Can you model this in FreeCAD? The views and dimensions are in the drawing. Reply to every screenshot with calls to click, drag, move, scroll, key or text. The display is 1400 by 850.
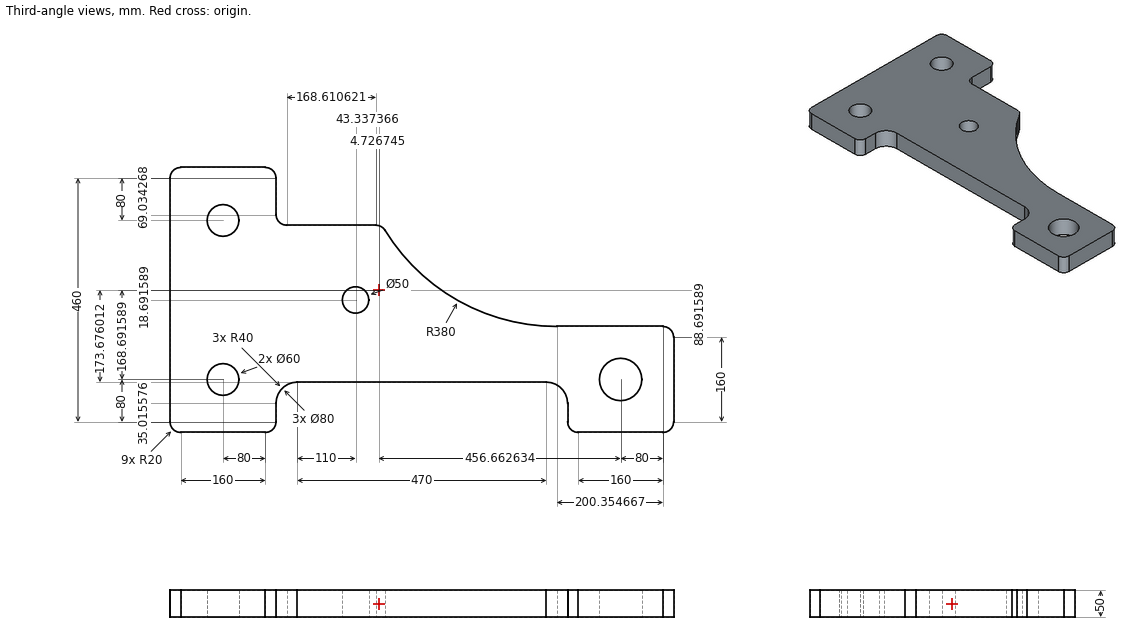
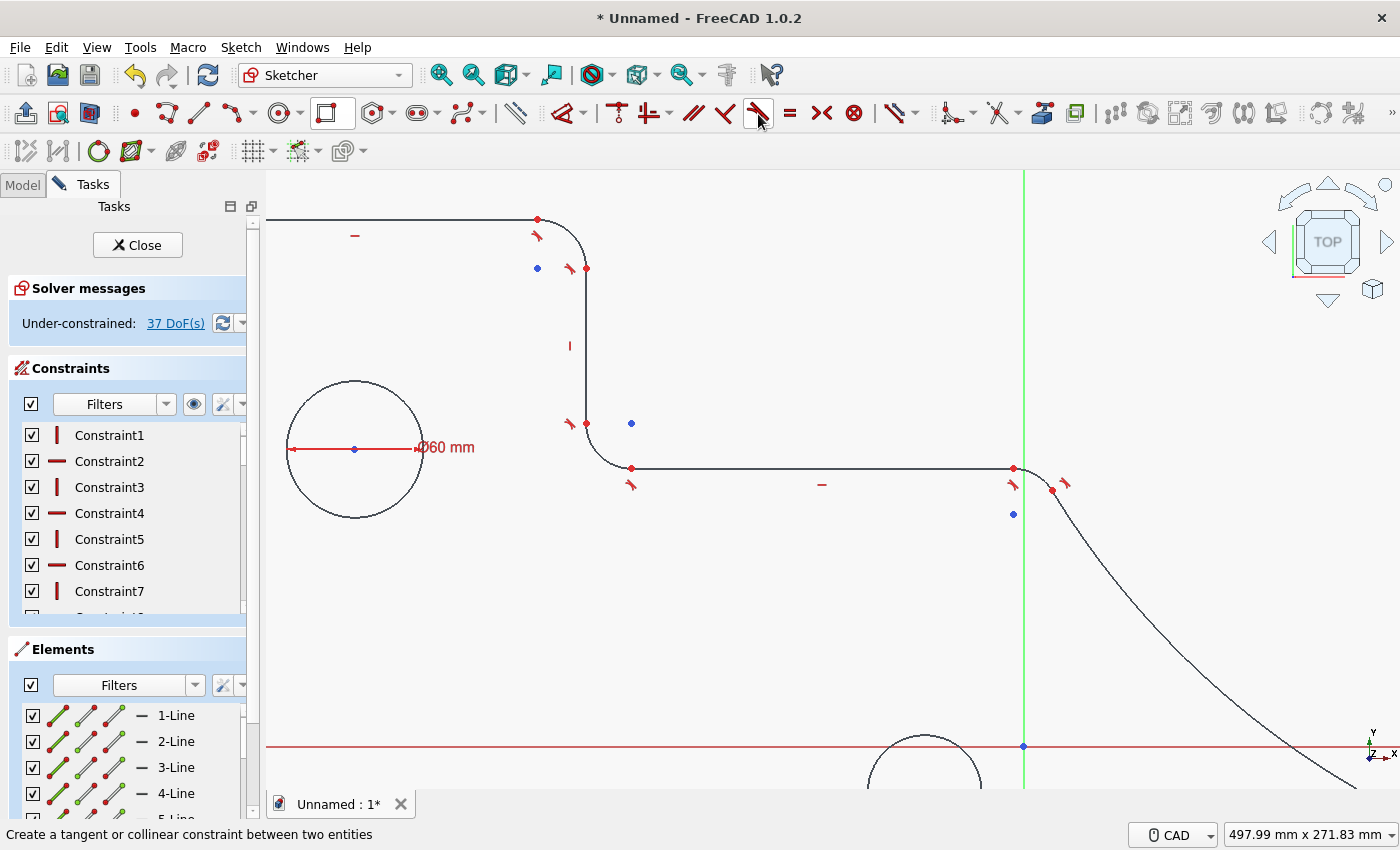
scroll(573, 346, down, 6)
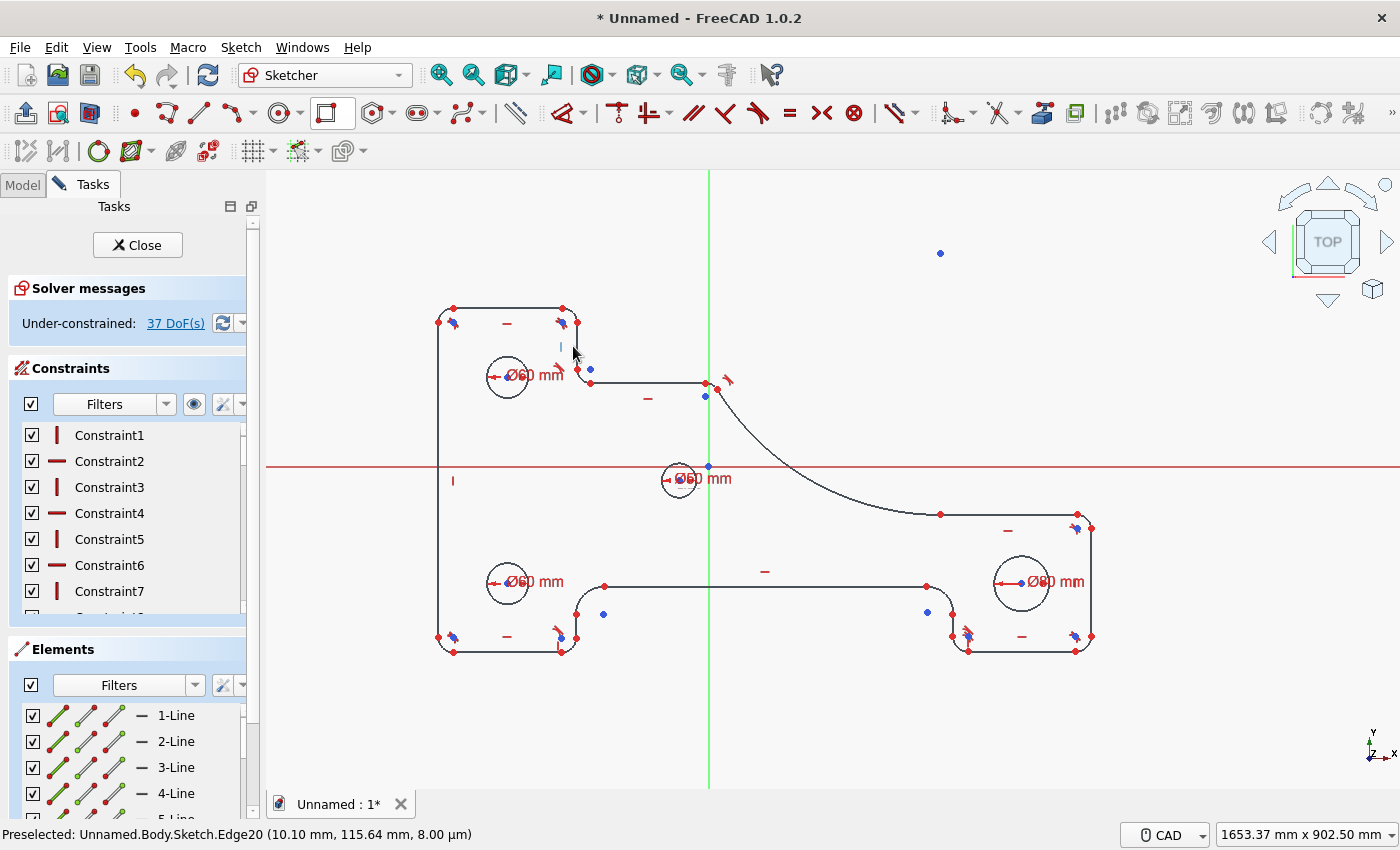
scroll(440, 644, up, 4)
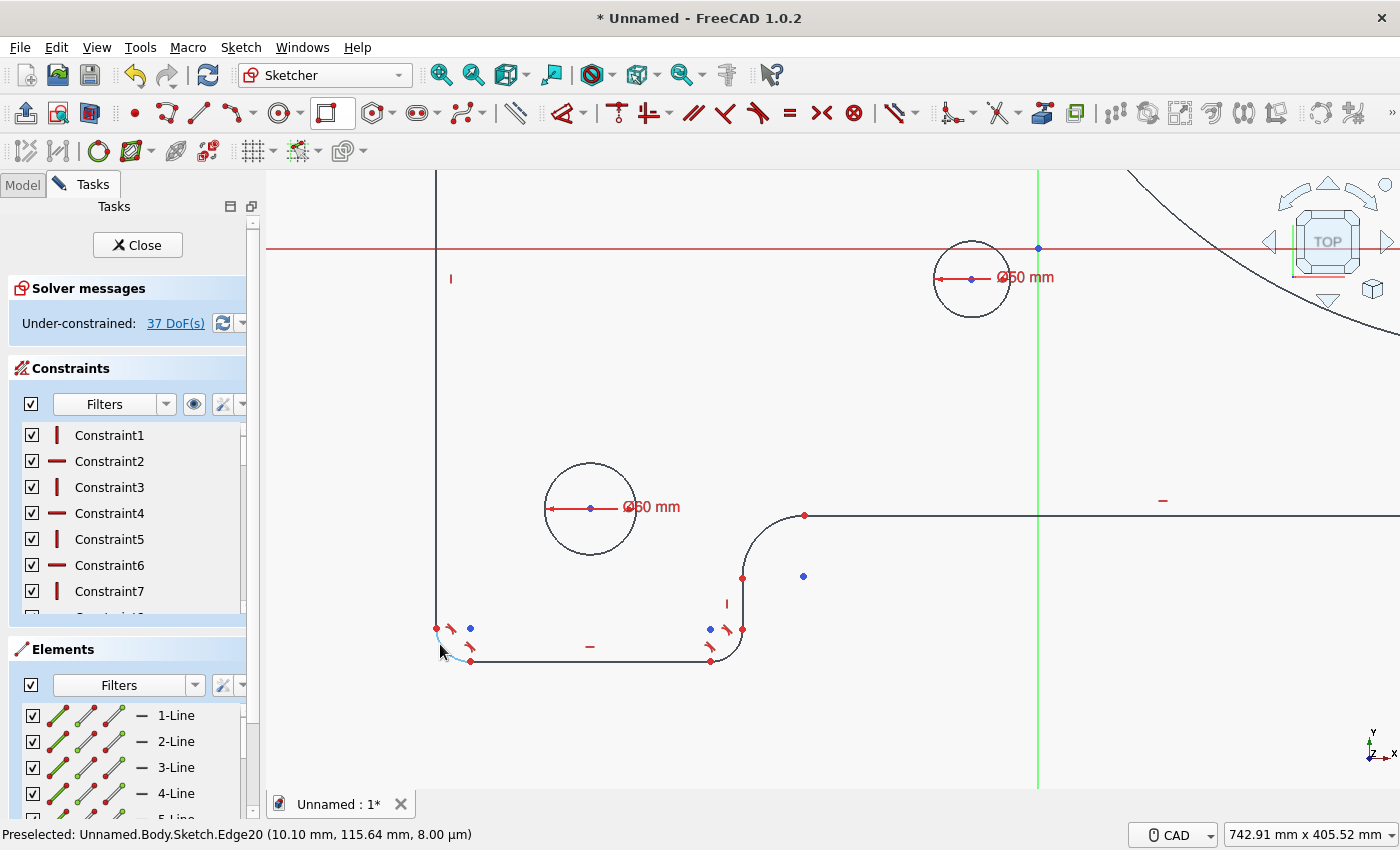
click(440, 643)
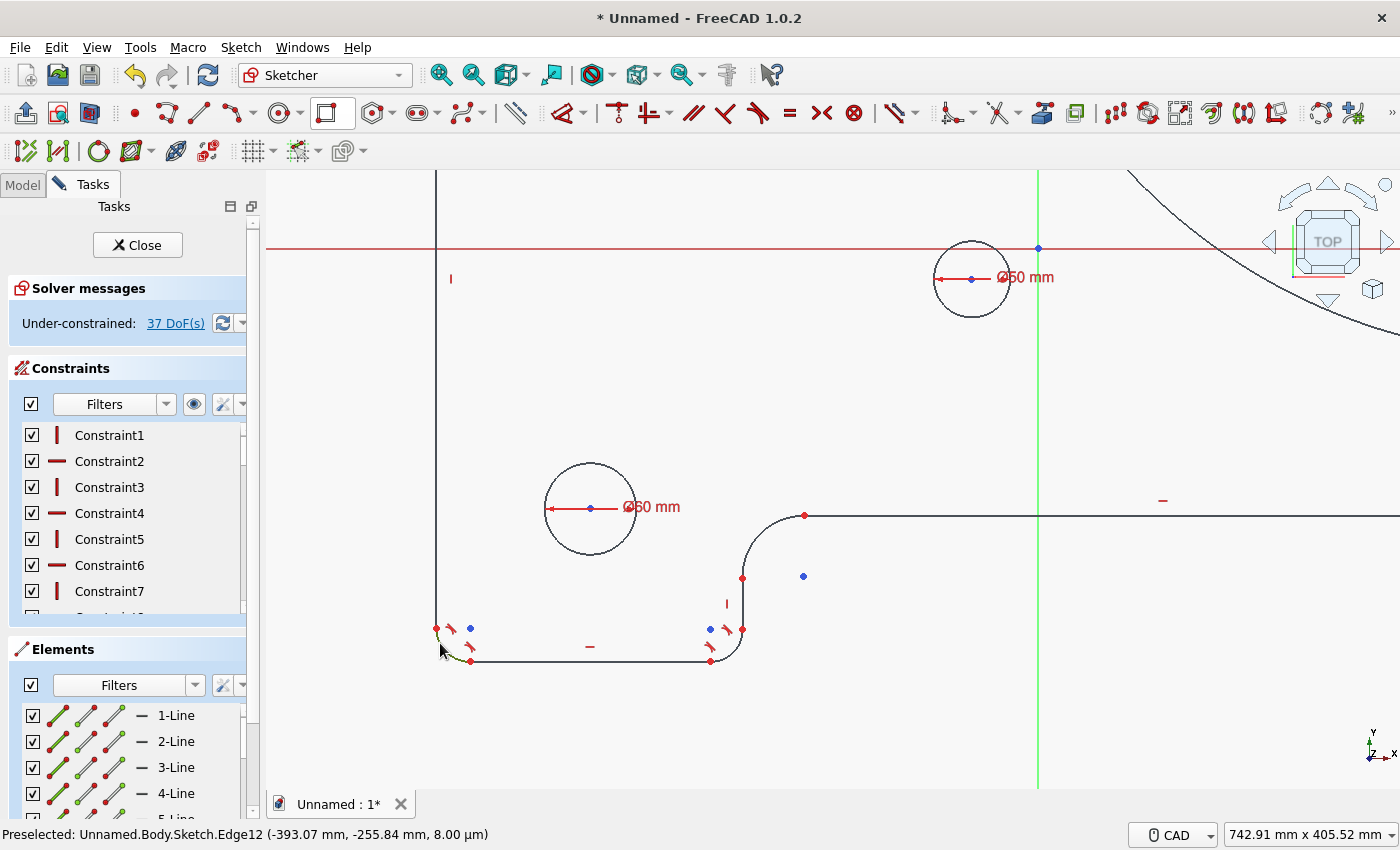
click(725, 658)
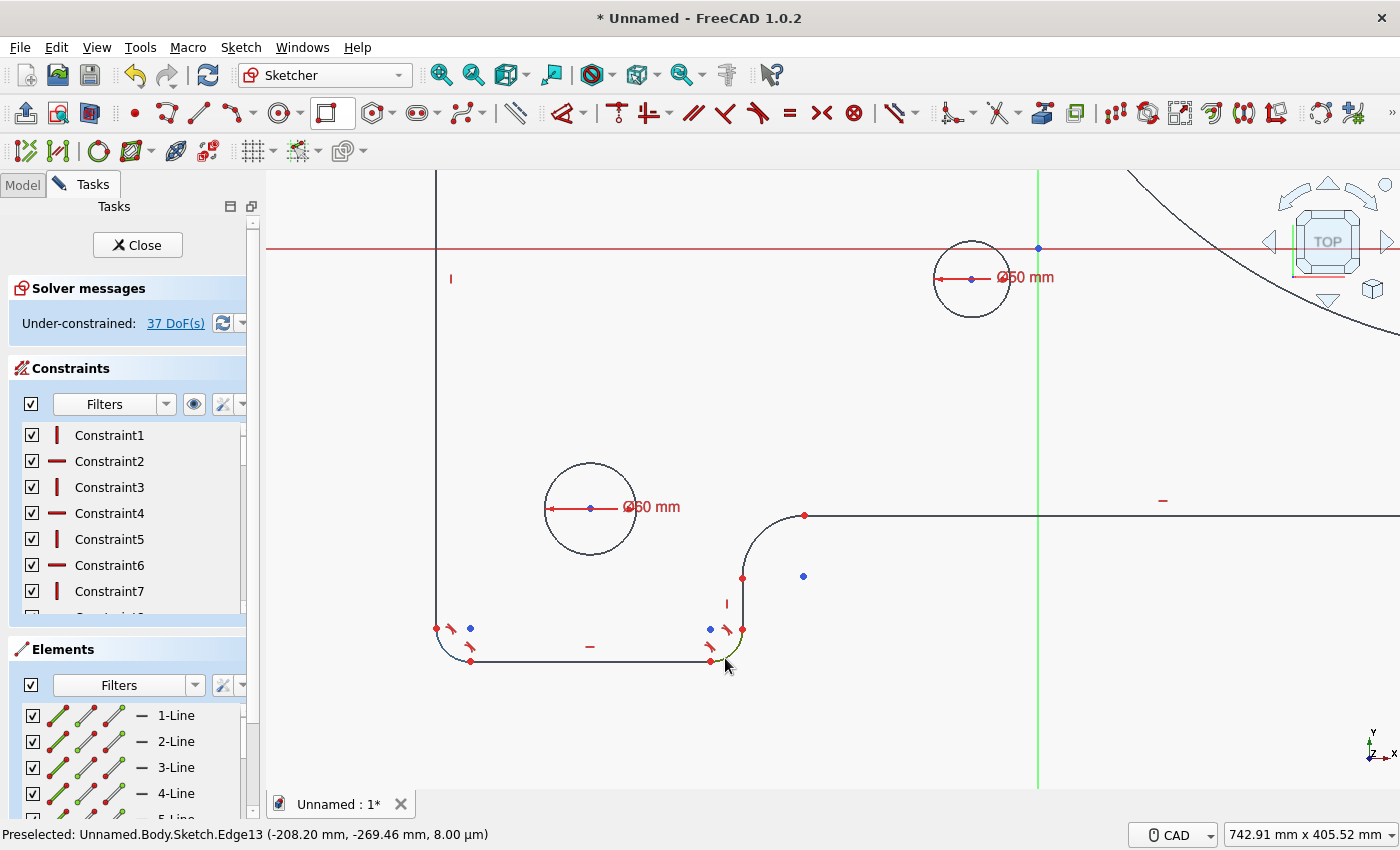
scroll(439, 644, down, 4)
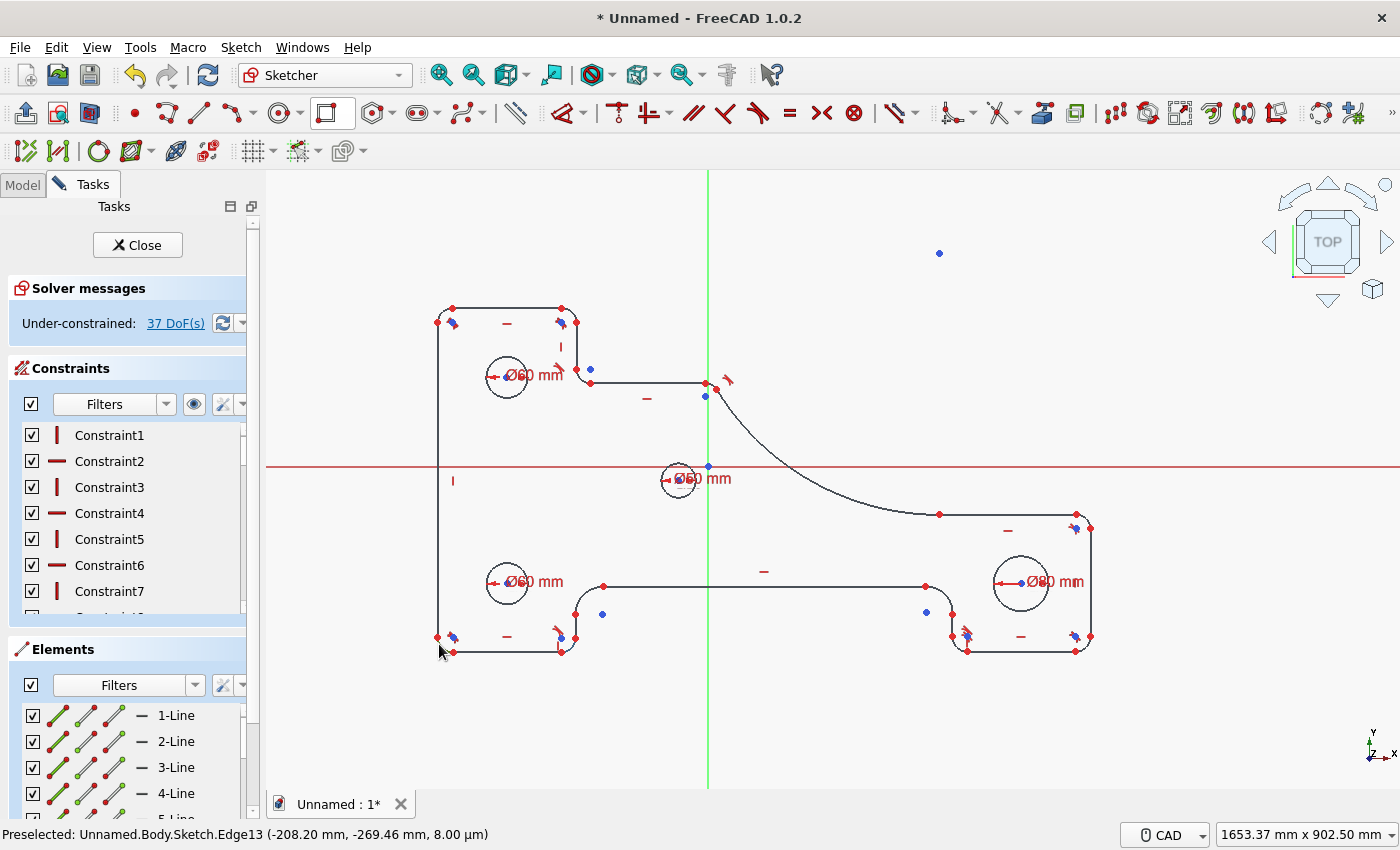
scroll(954, 643, up, 4)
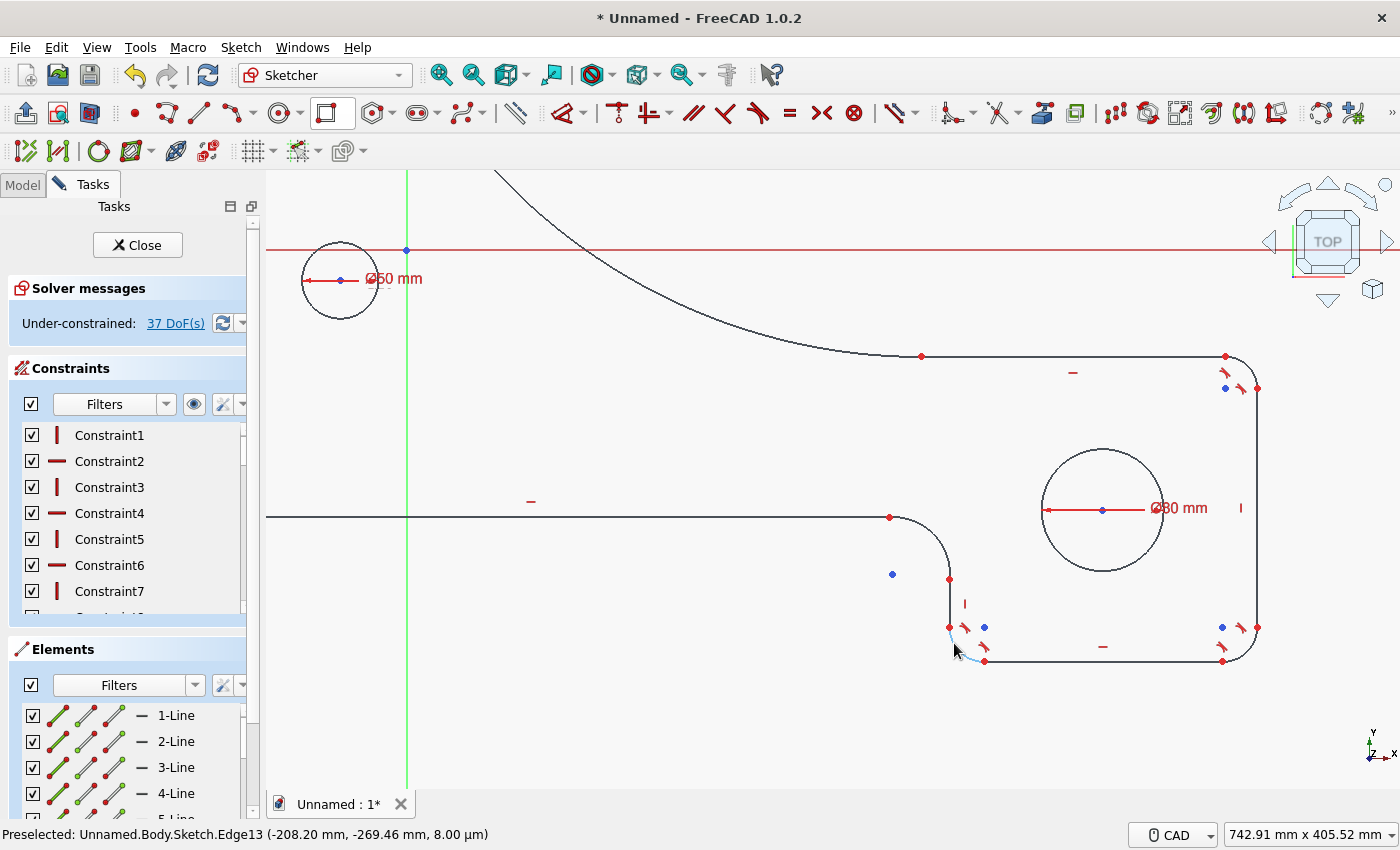
click(953, 643)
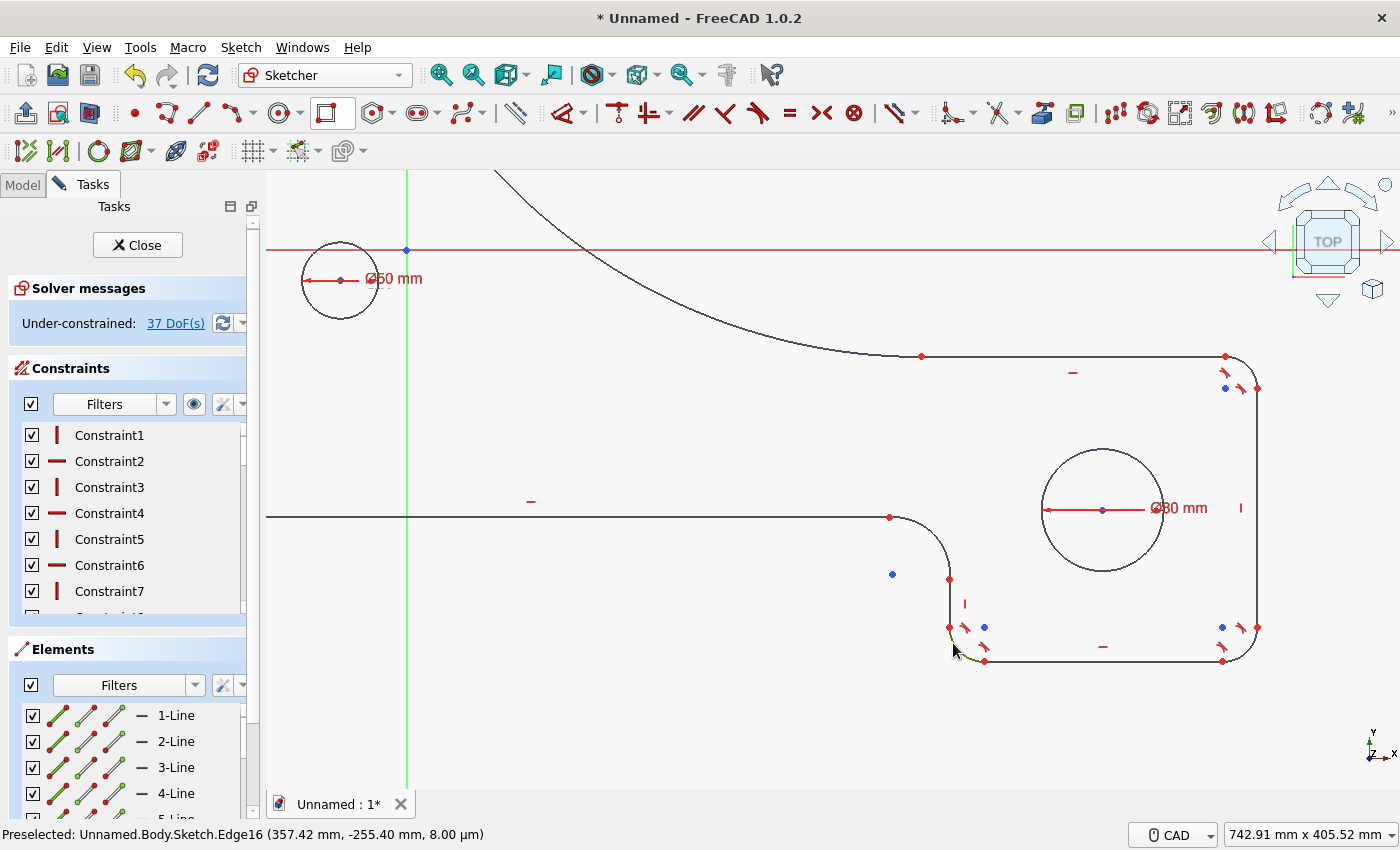
scroll(1233, 660, up, 2)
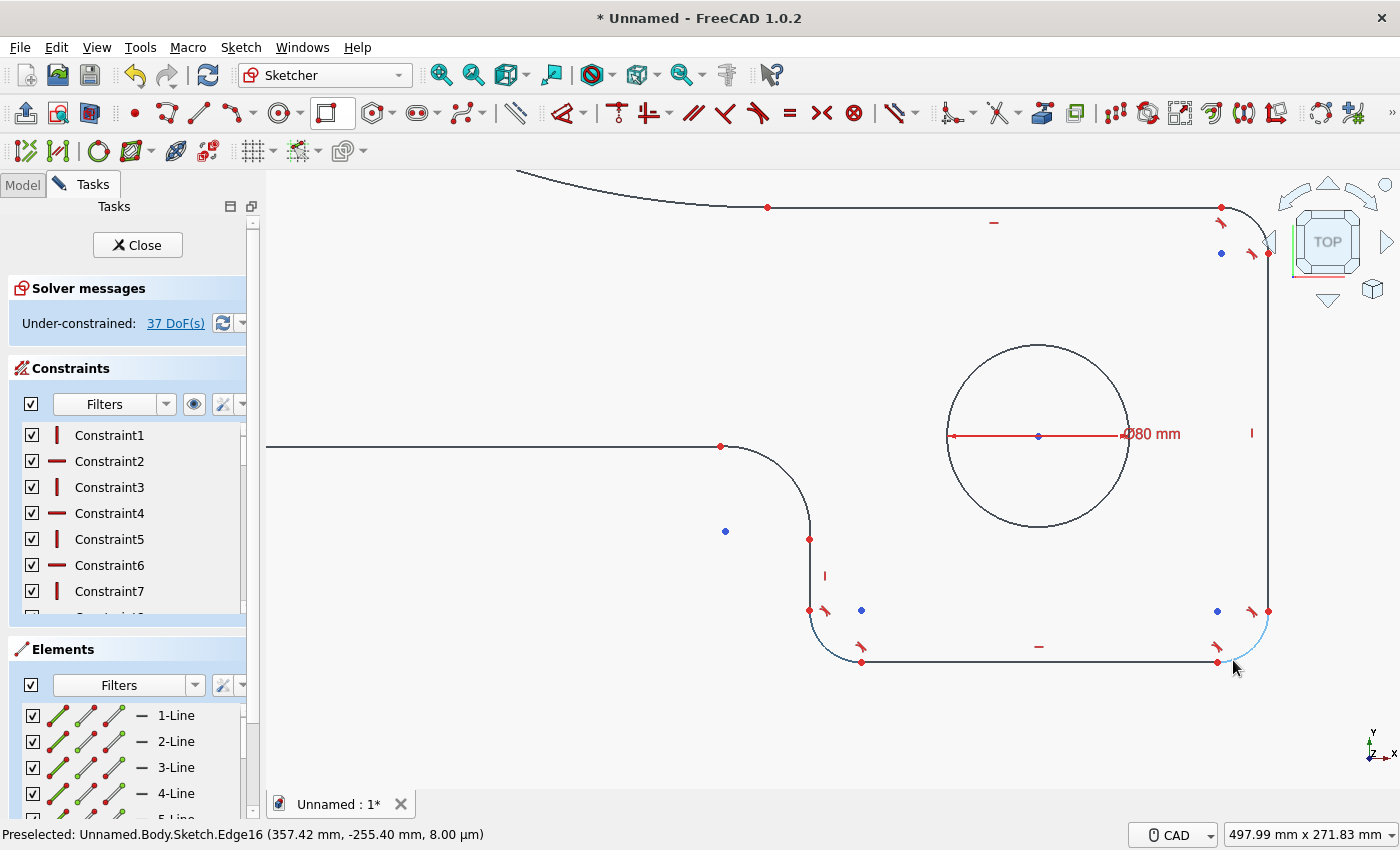
click(1233, 660)